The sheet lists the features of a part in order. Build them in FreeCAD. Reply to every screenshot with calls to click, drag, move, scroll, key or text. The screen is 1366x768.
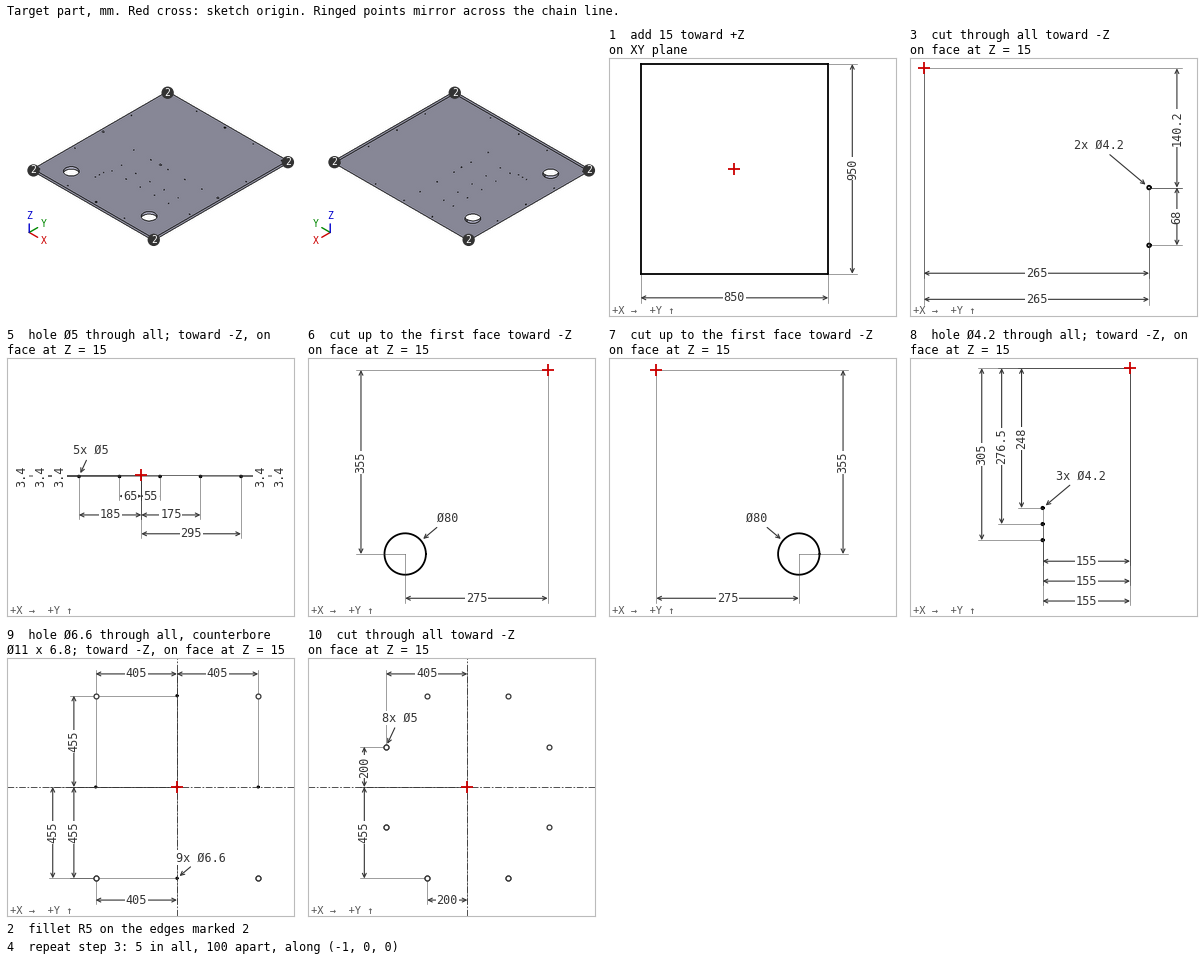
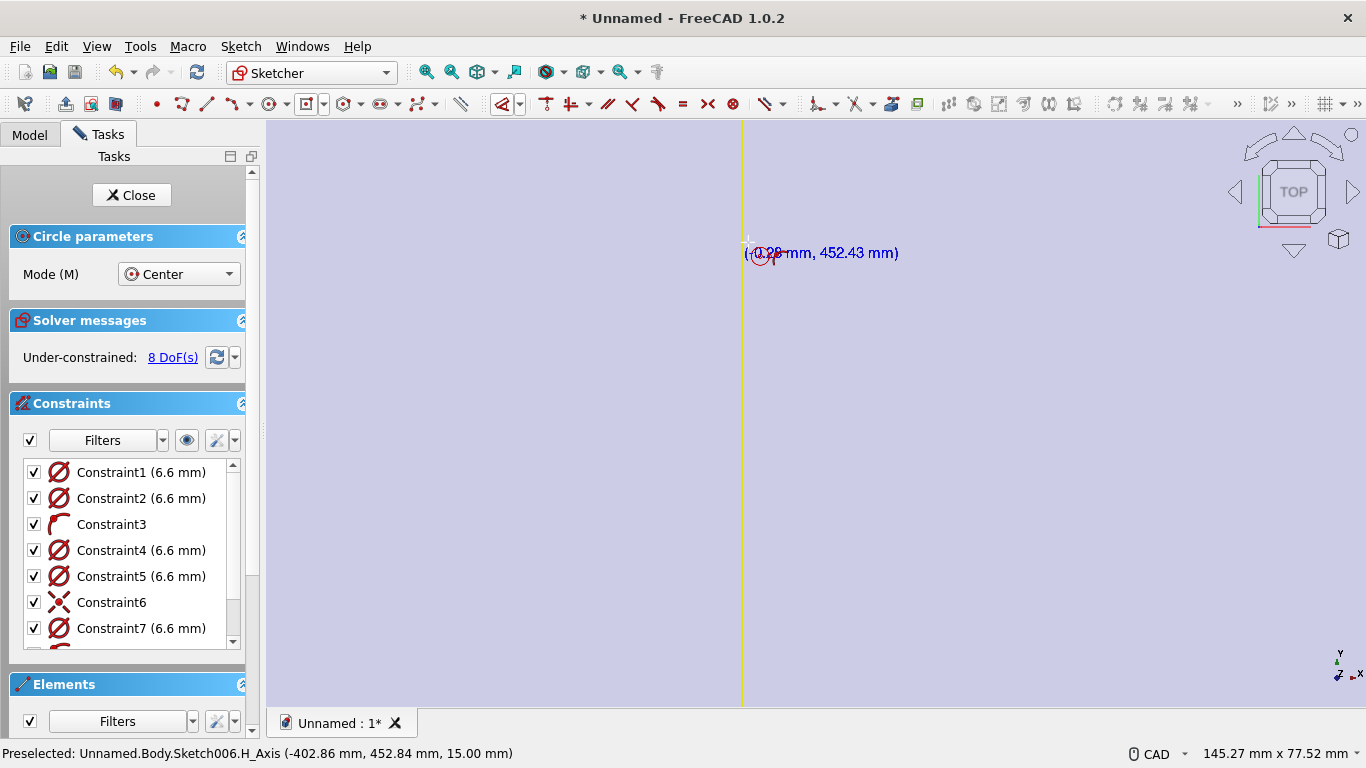
scroll(748, 242, down, 15)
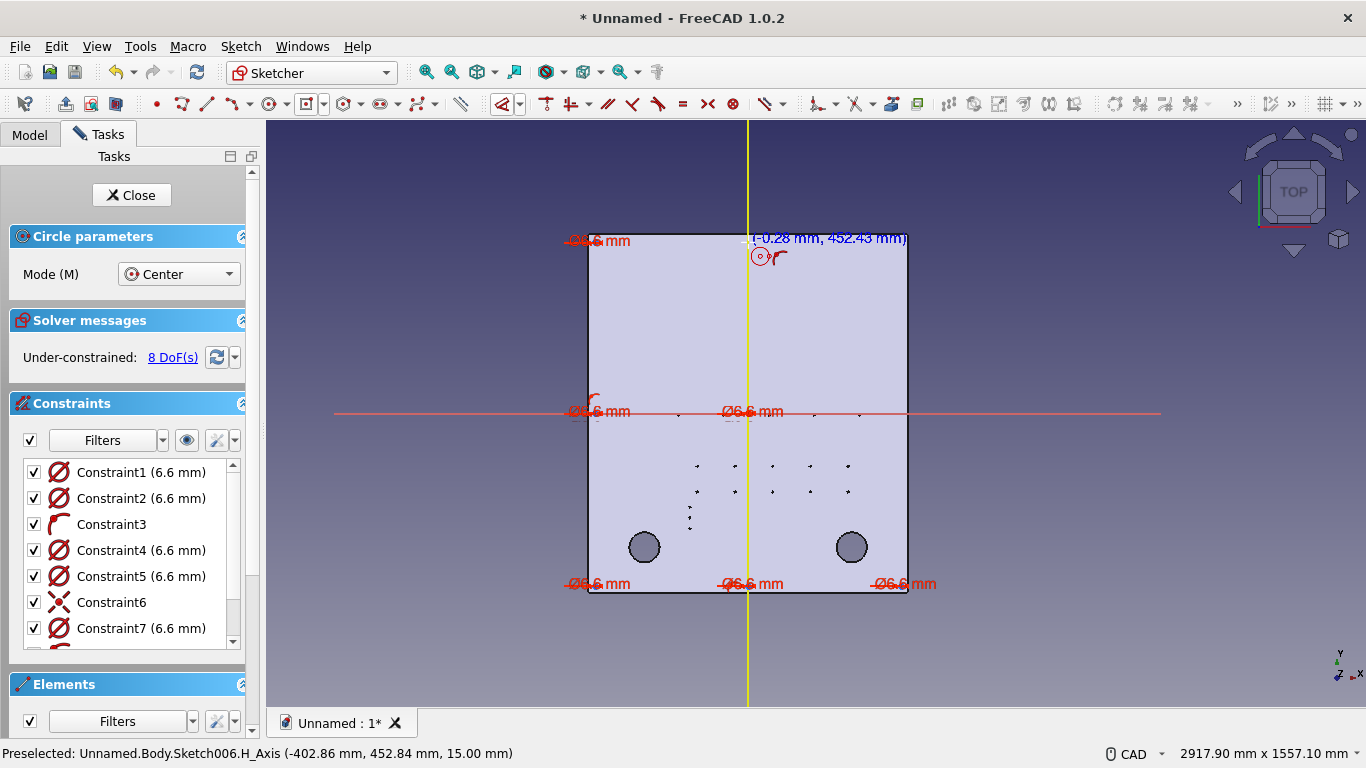
click(748, 242)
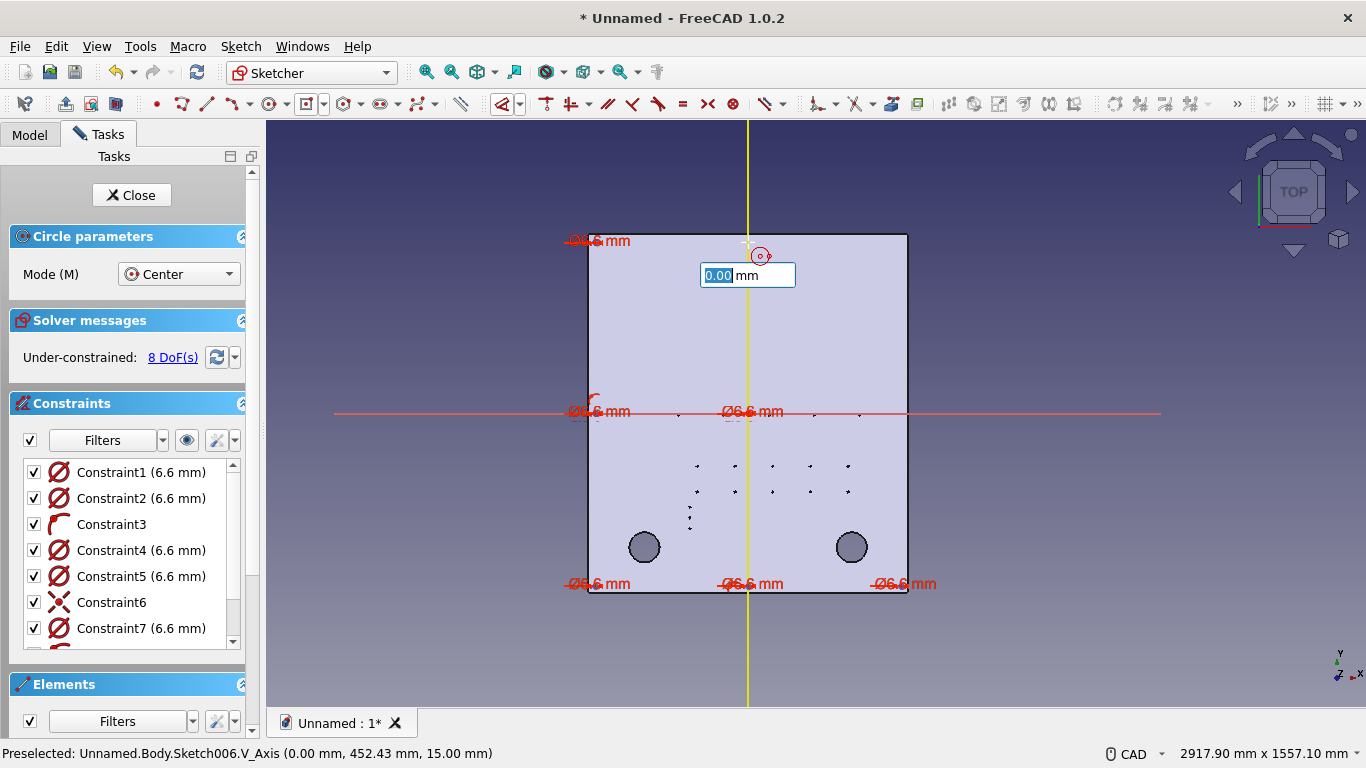
scroll(749, 242, up, 14)
move(747, 232)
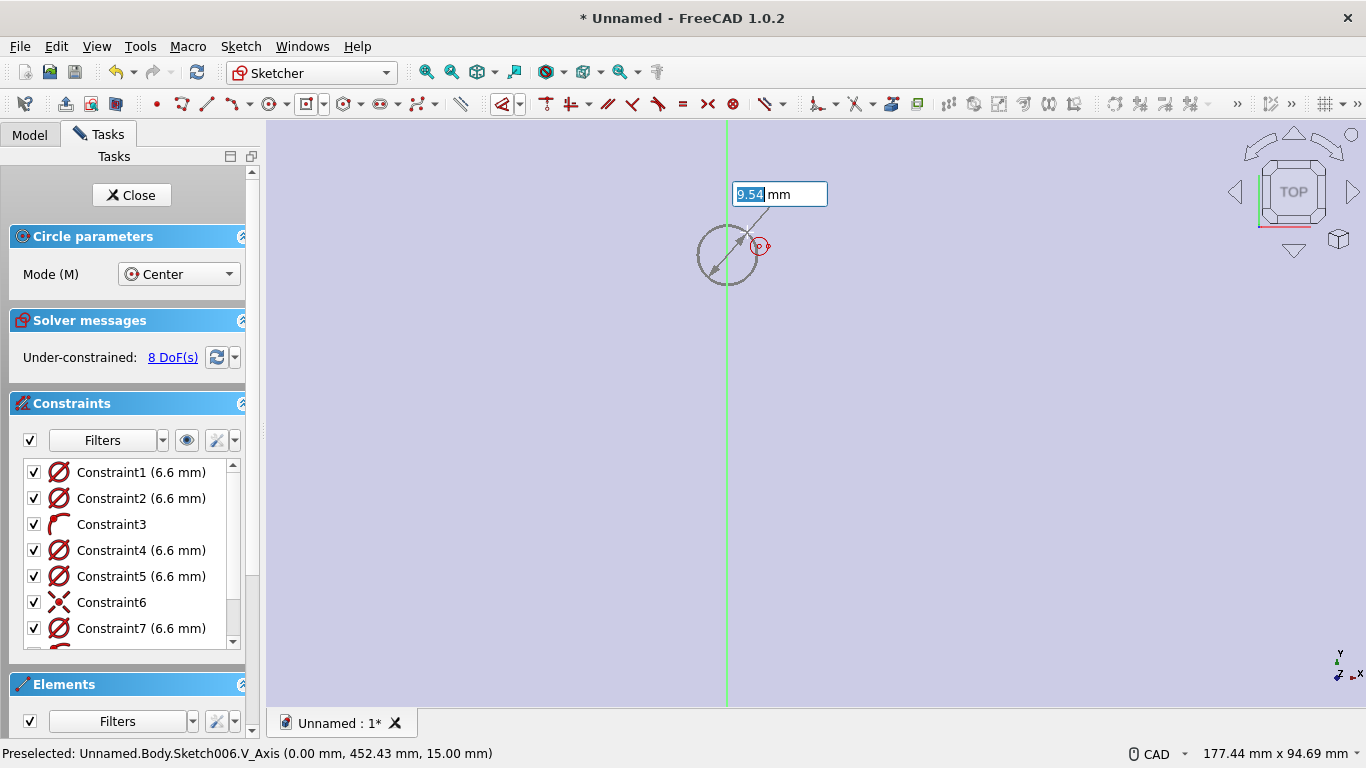
text(6.6)
key(Return)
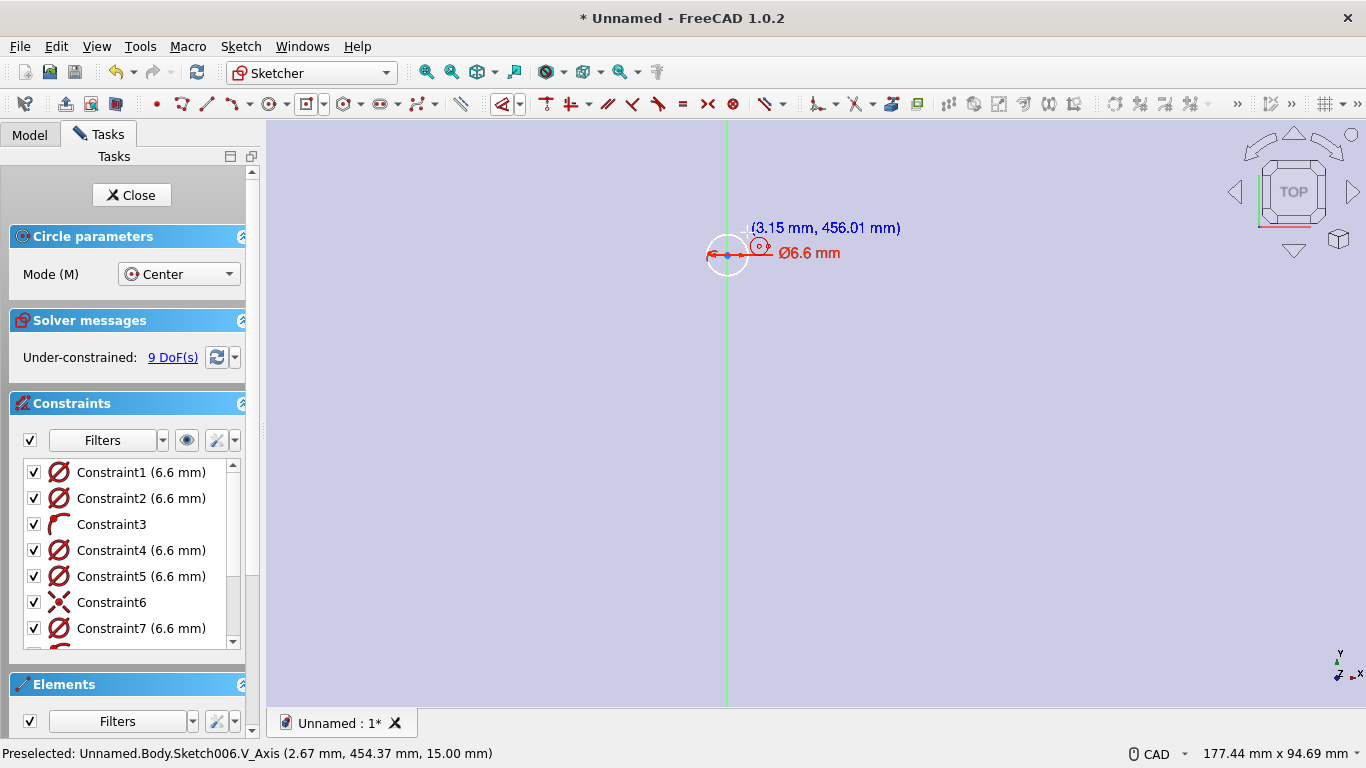
scroll(749, 242, down, 14)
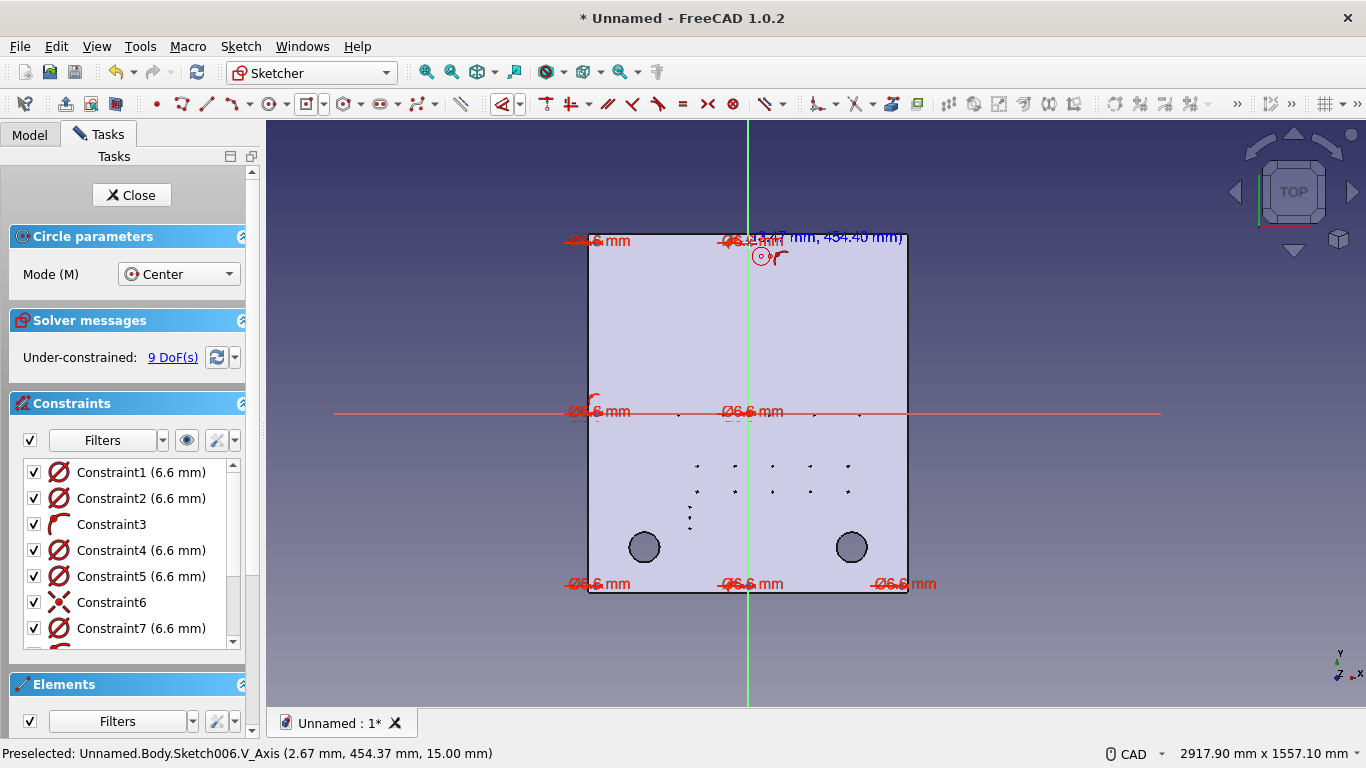
scroll(901, 242, up, 15)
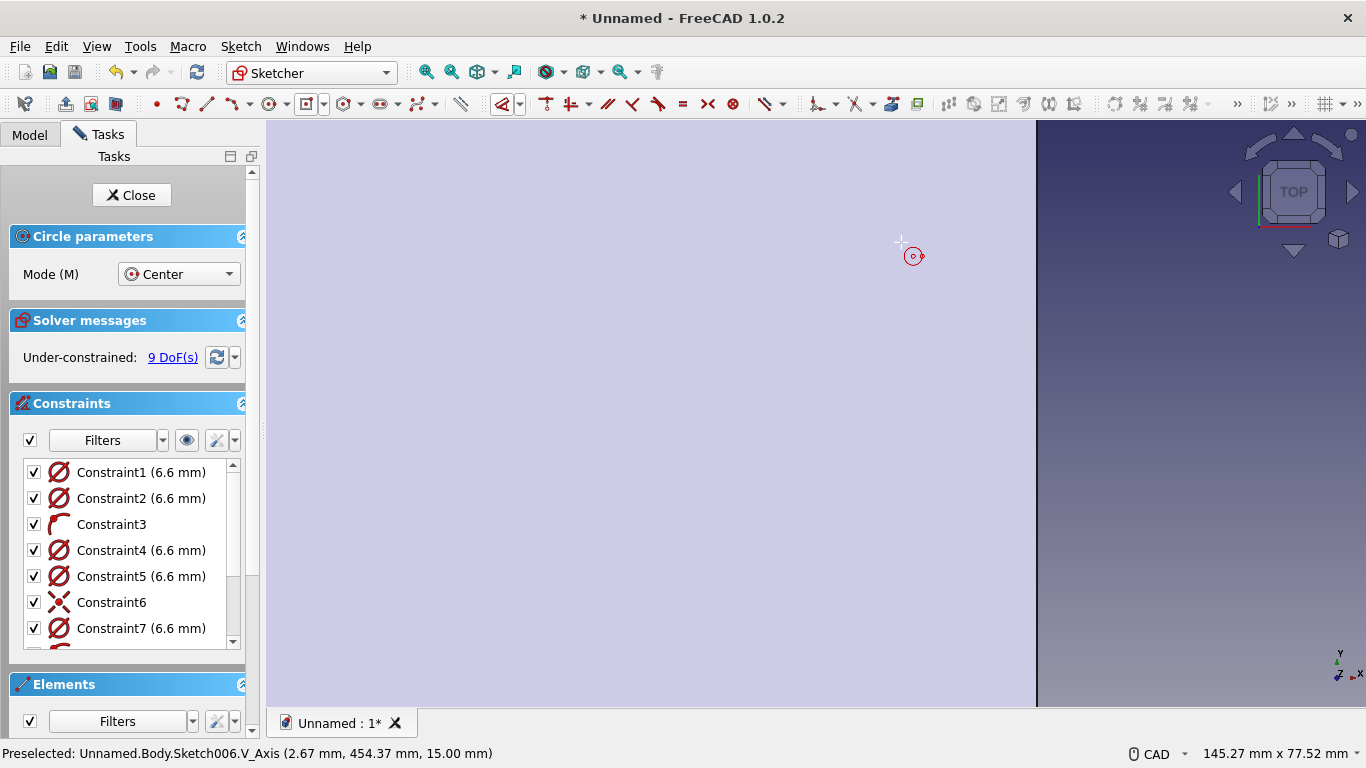
scroll(901, 242, down, 15)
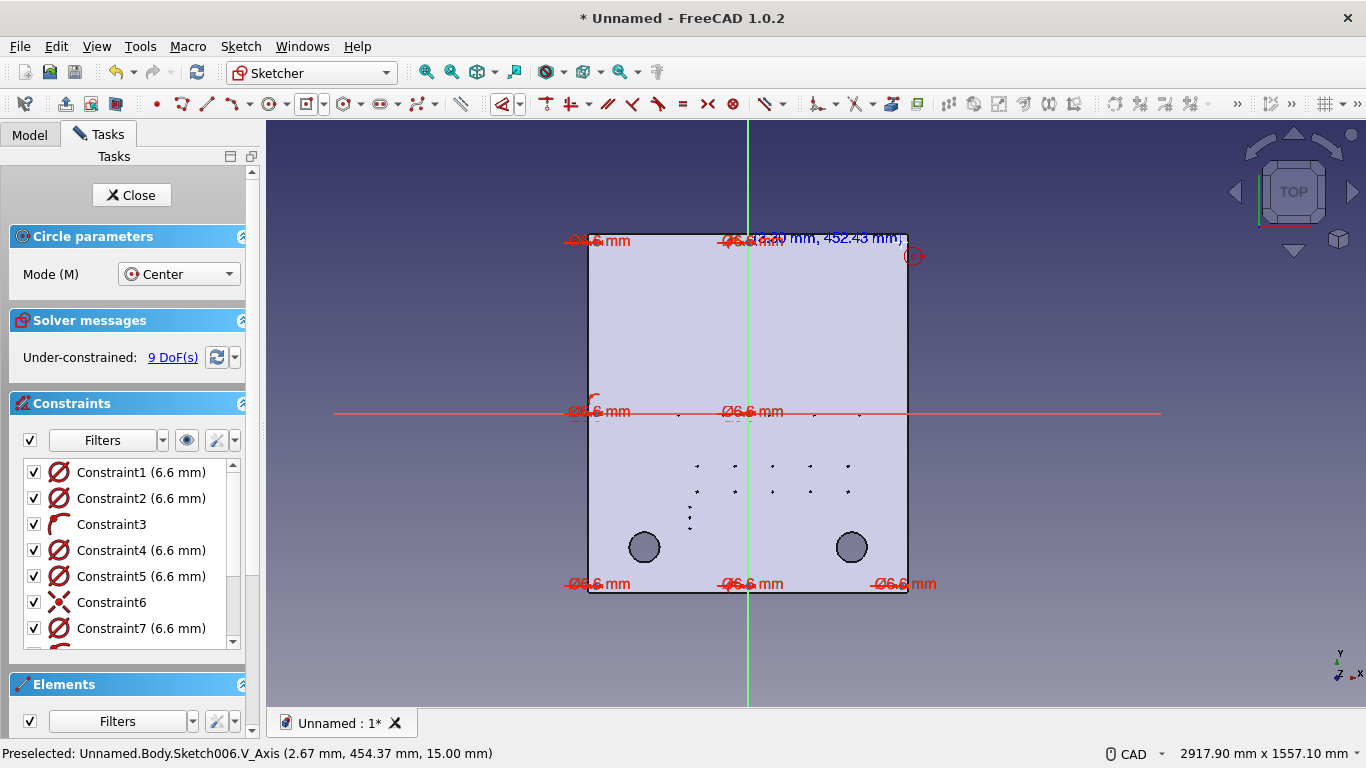
click(901, 242)
move(902, 241)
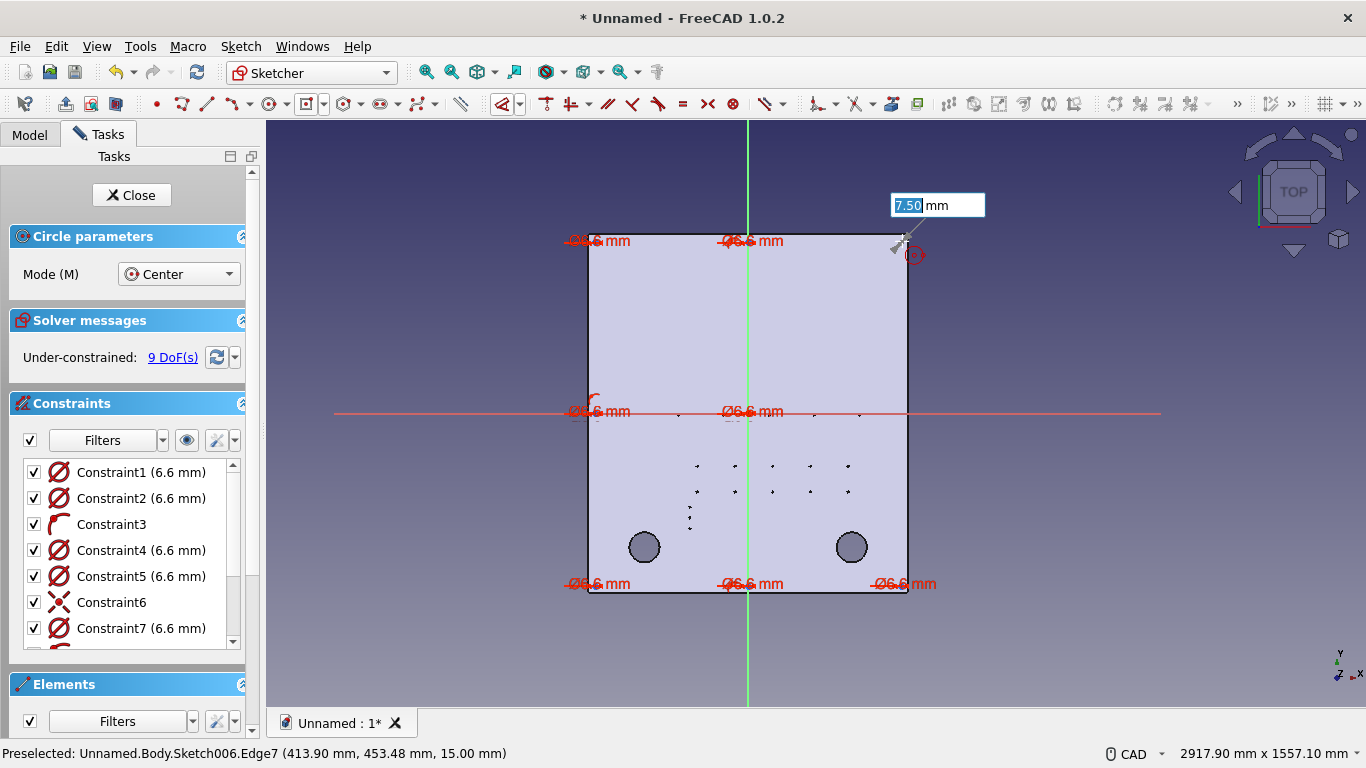
text(6.6)
key(Return)